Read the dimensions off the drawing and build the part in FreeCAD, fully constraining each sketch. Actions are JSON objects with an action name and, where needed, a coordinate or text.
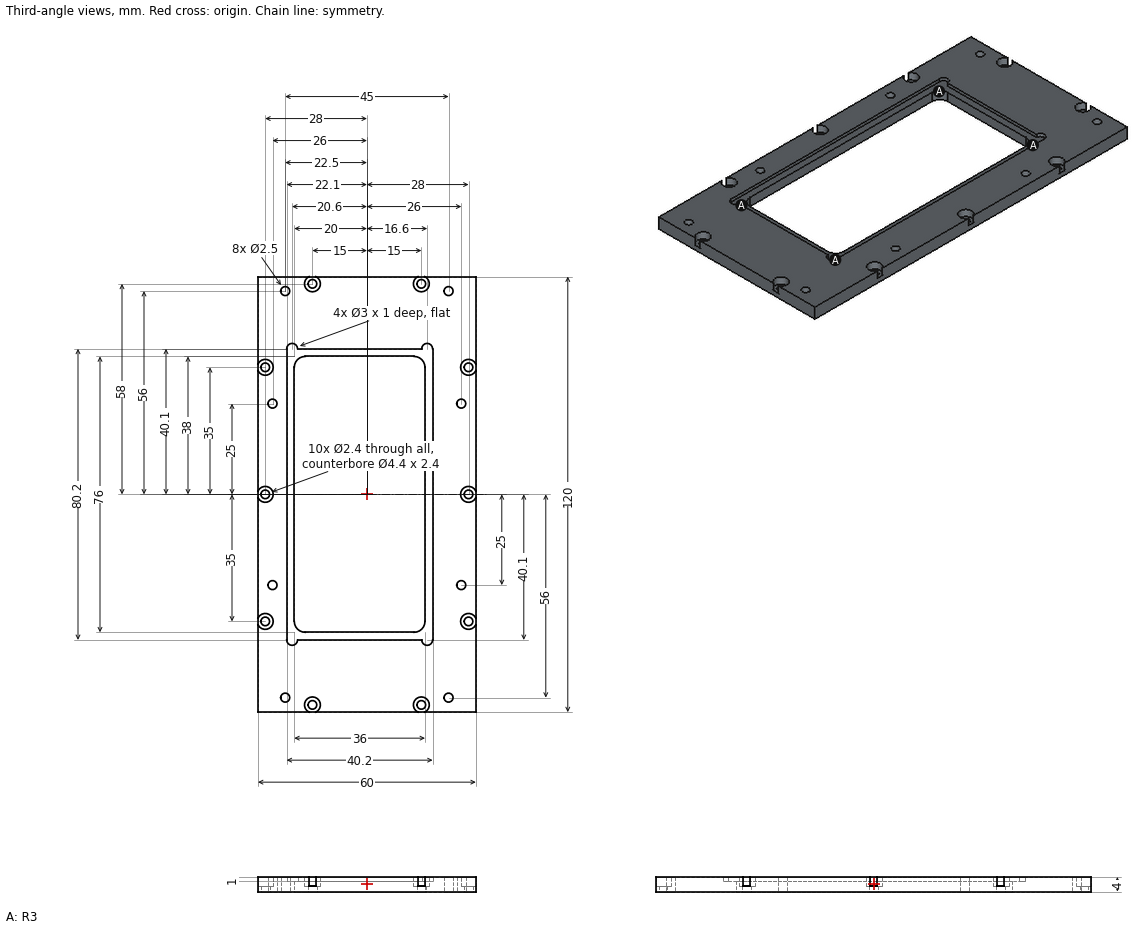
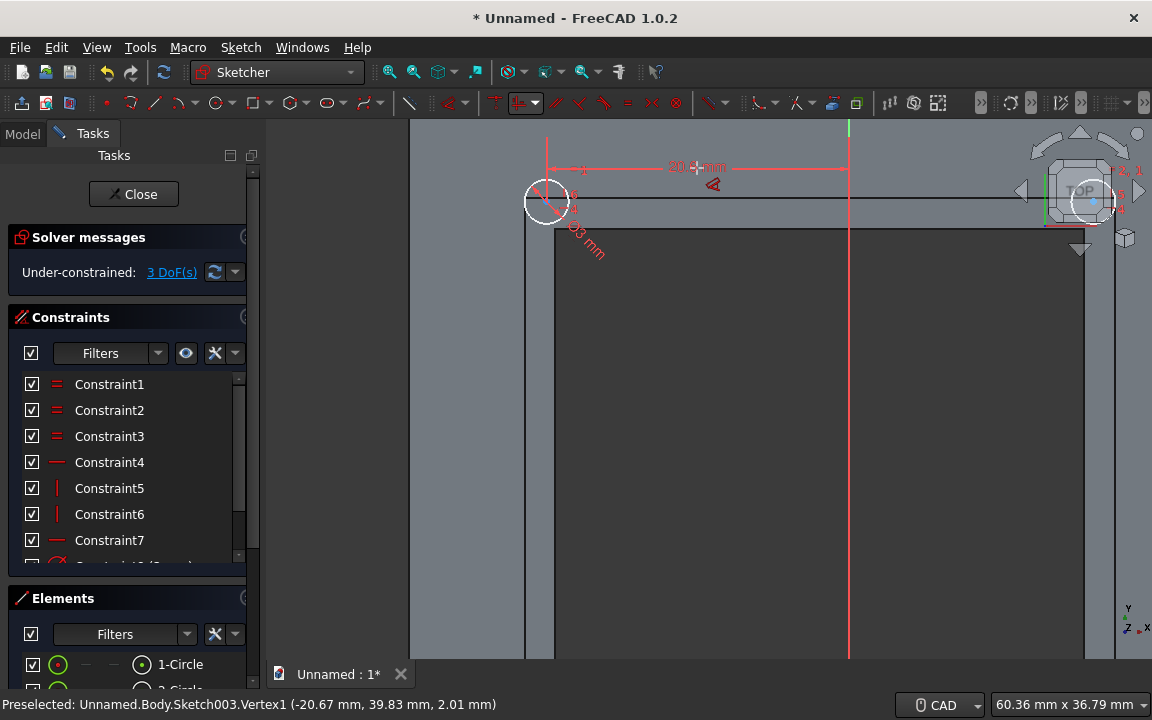
{"action": "left_click", "coordinate": [547, 202]}
{"action": "left_click", "coordinate": [513, 416]}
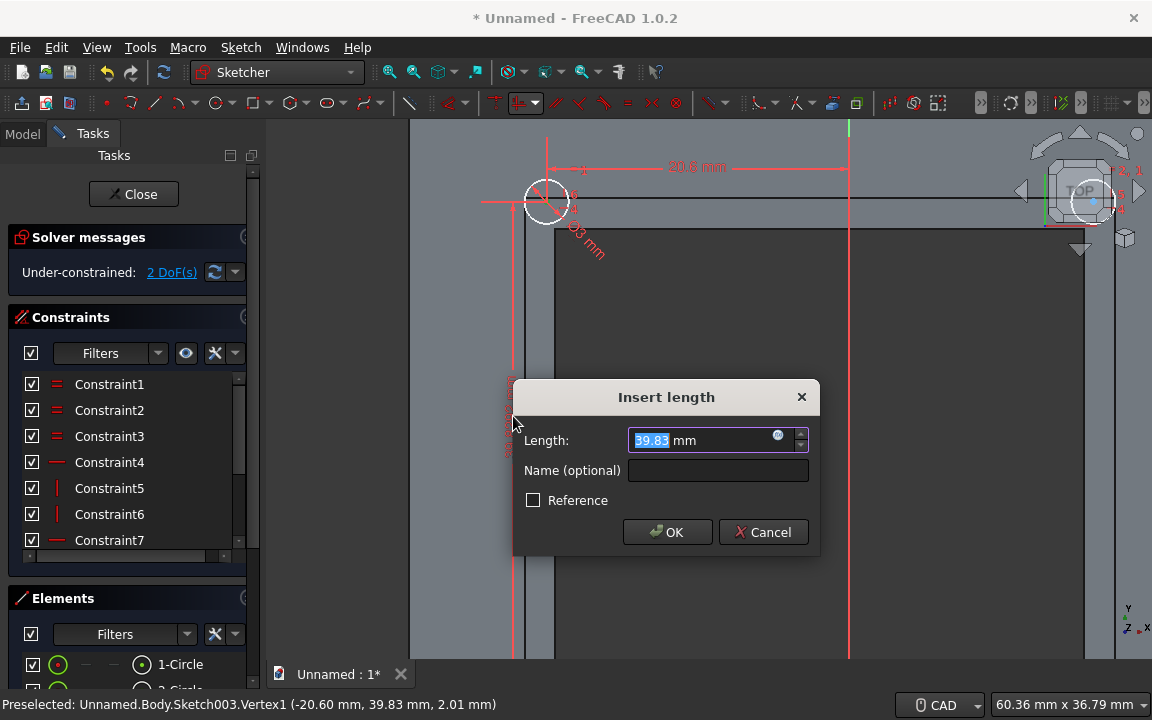
{"action": "type", "text": "40.1"}
{"action": "key", "text": "Return"}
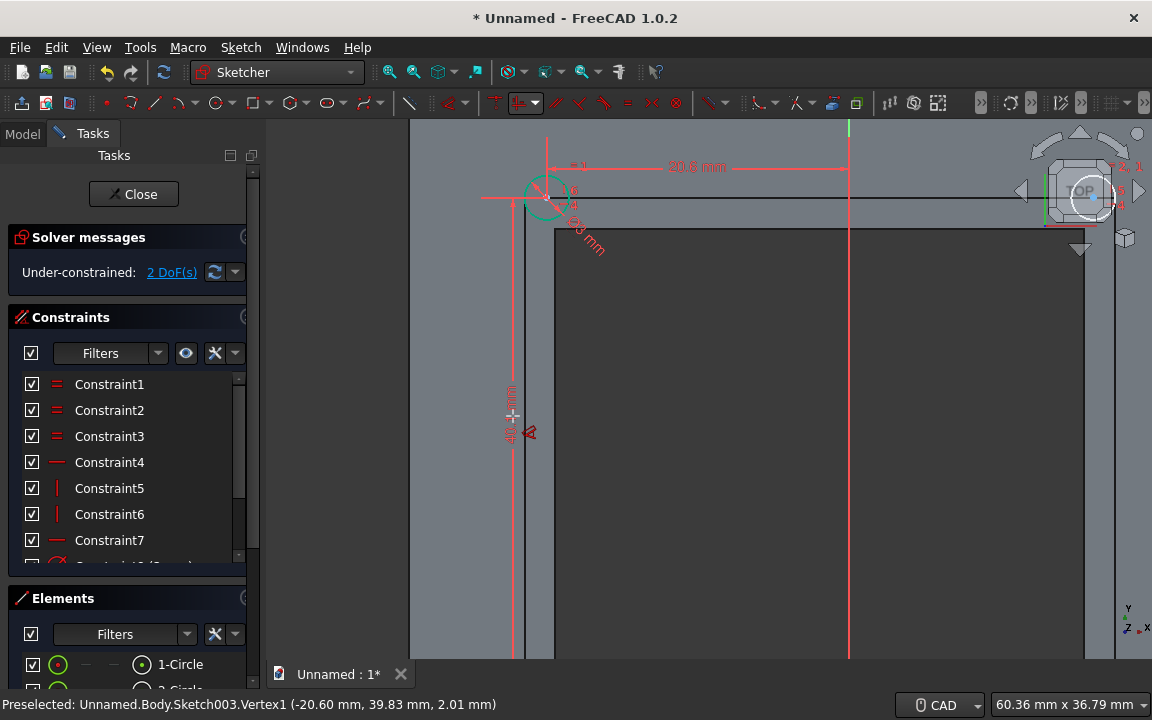
{"action": "scroll", "coordinate": [563, 218], "scroll_direction": "down", "scroll_amount": 6}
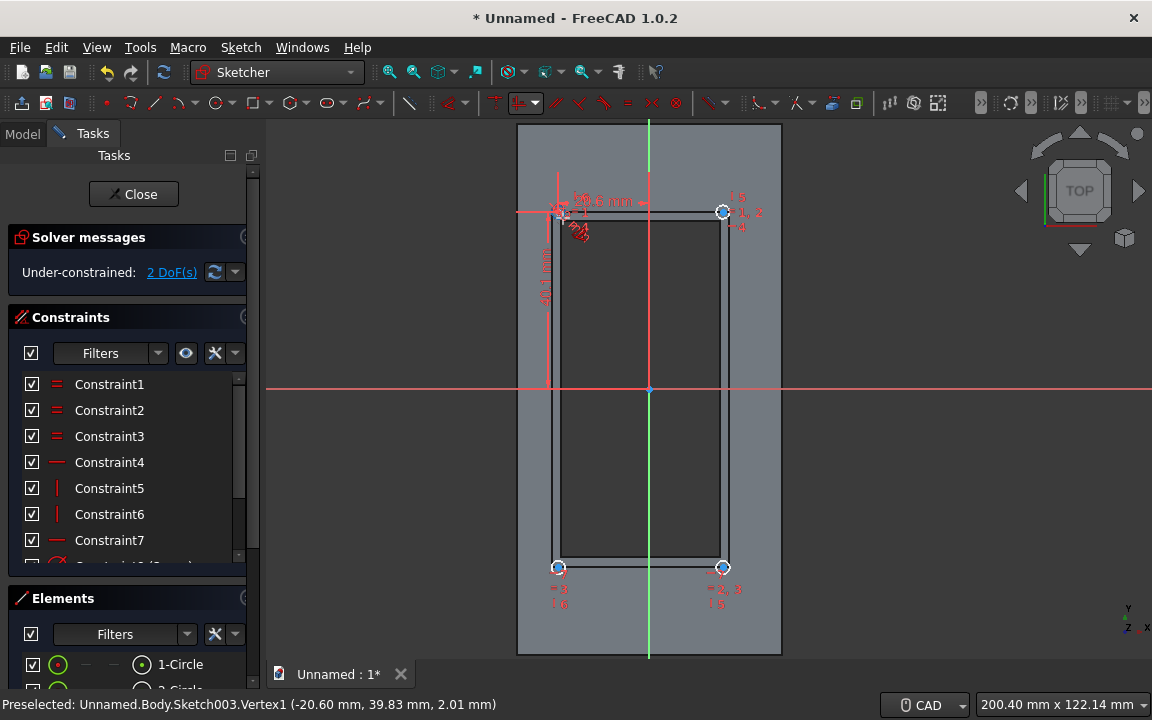
{"action": "left_click", "coordinate": [723, 212]}
{"action": "left_click", "coordinate": [686, 178]}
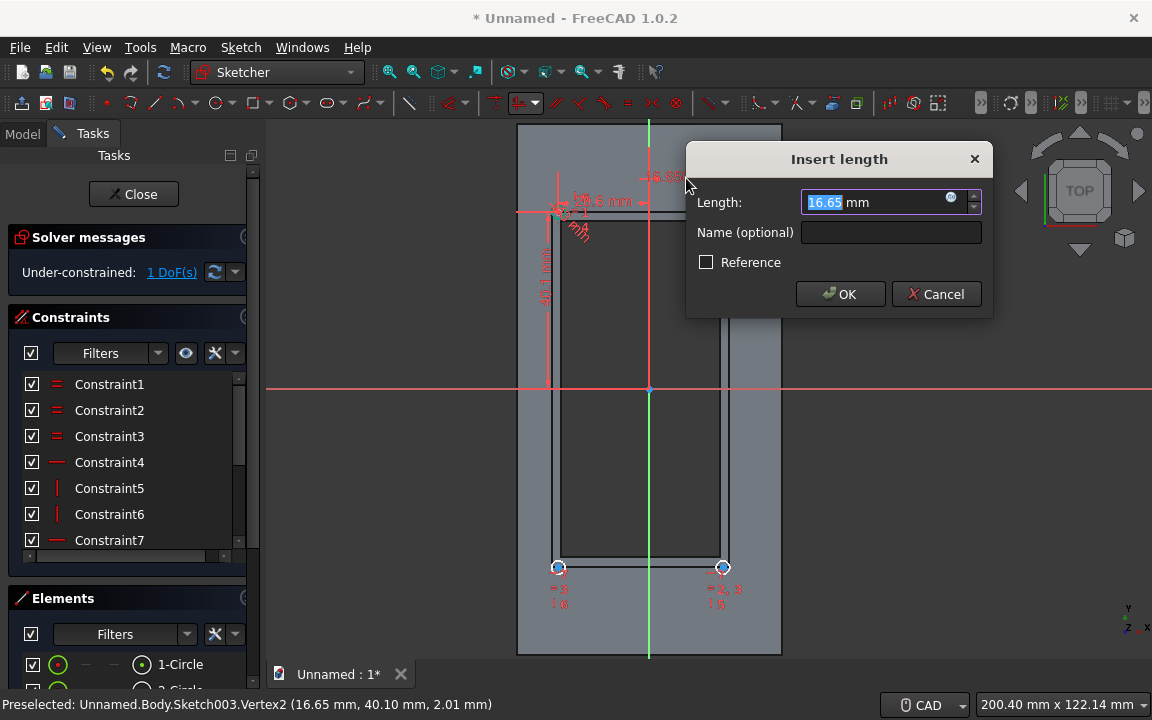
{"action": "type", "text": "16.6"}
{"action": "key", "text": "Return"}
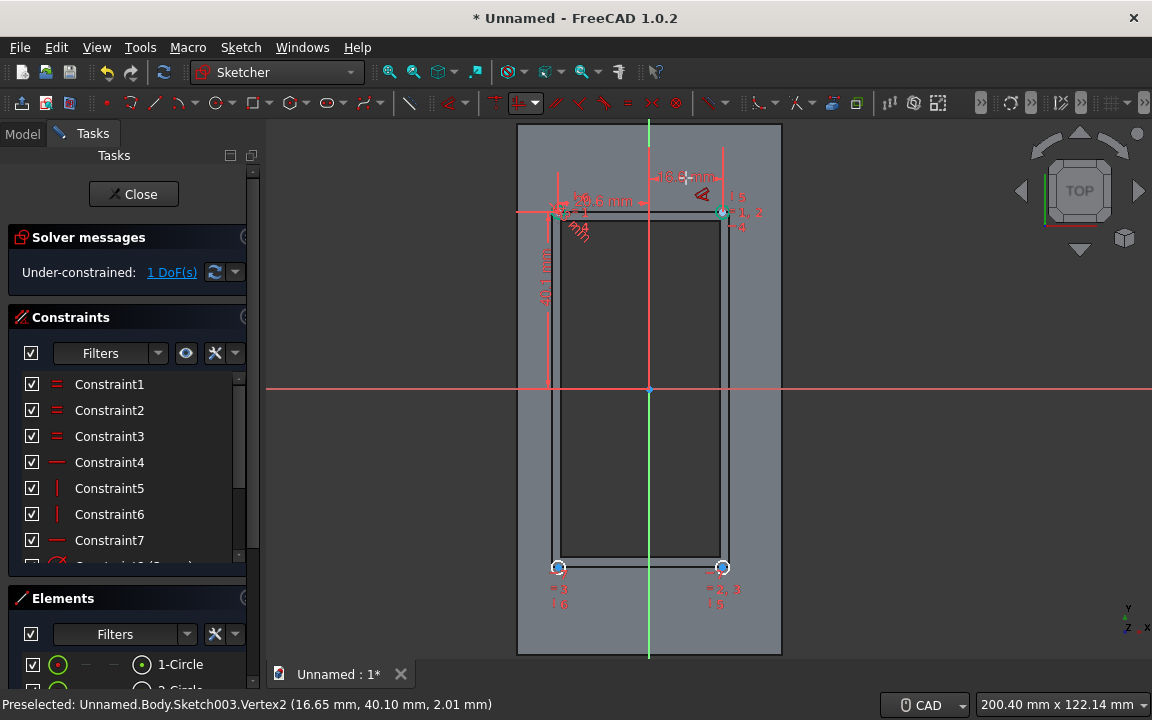
{"action": "left_click", "coordinate": [723, 567]}
{"action": "left_click", "coordinate": [757, 478]}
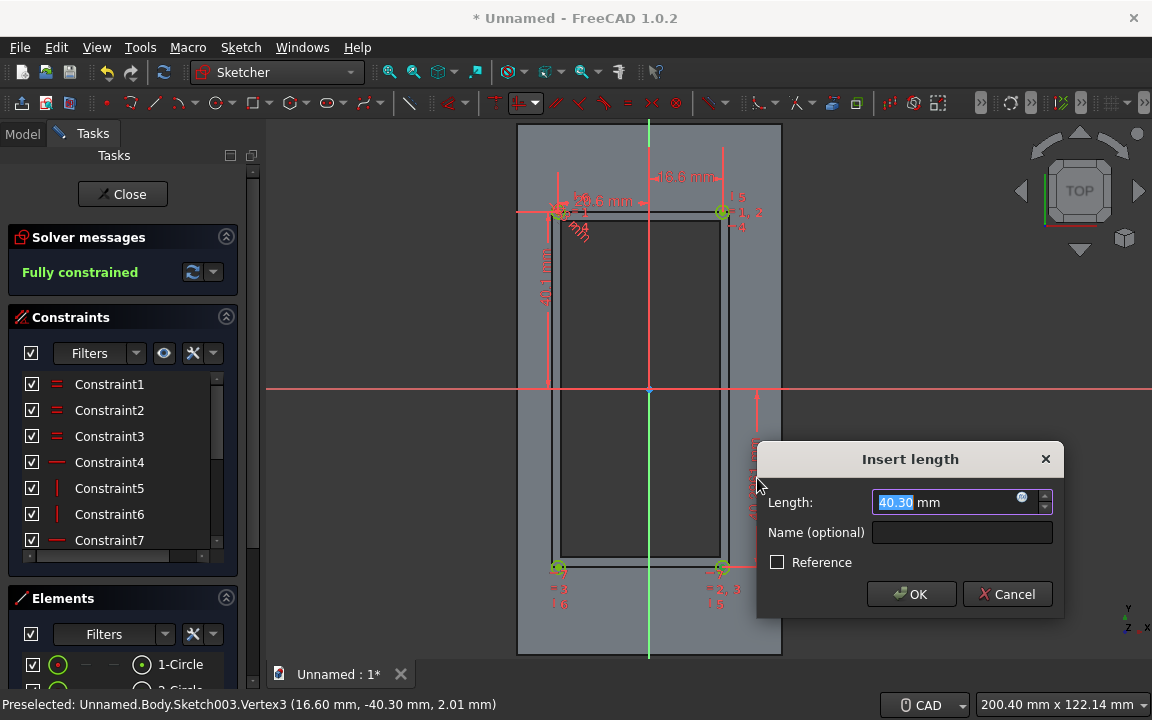
{"action": "type", "text": "40.1"}
{"action": "key", "text": "Return"}
{"action": "key", "text": "Escape"}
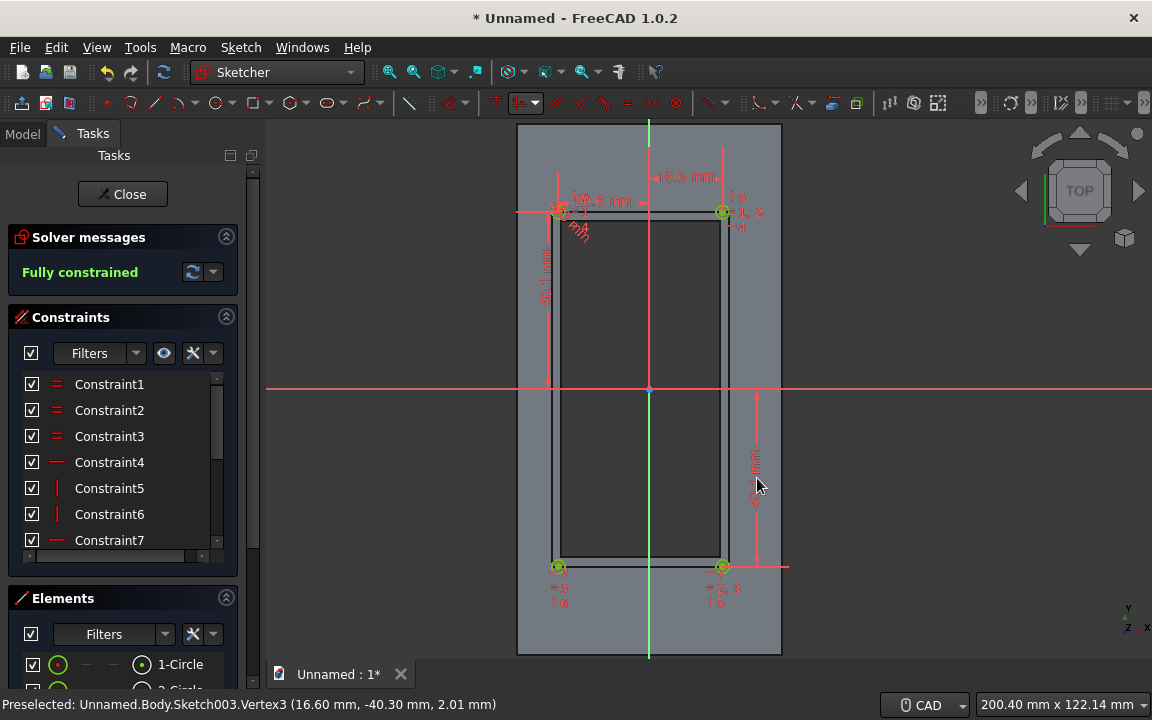
{"action": "left_click", "coordinate": [123, 194]}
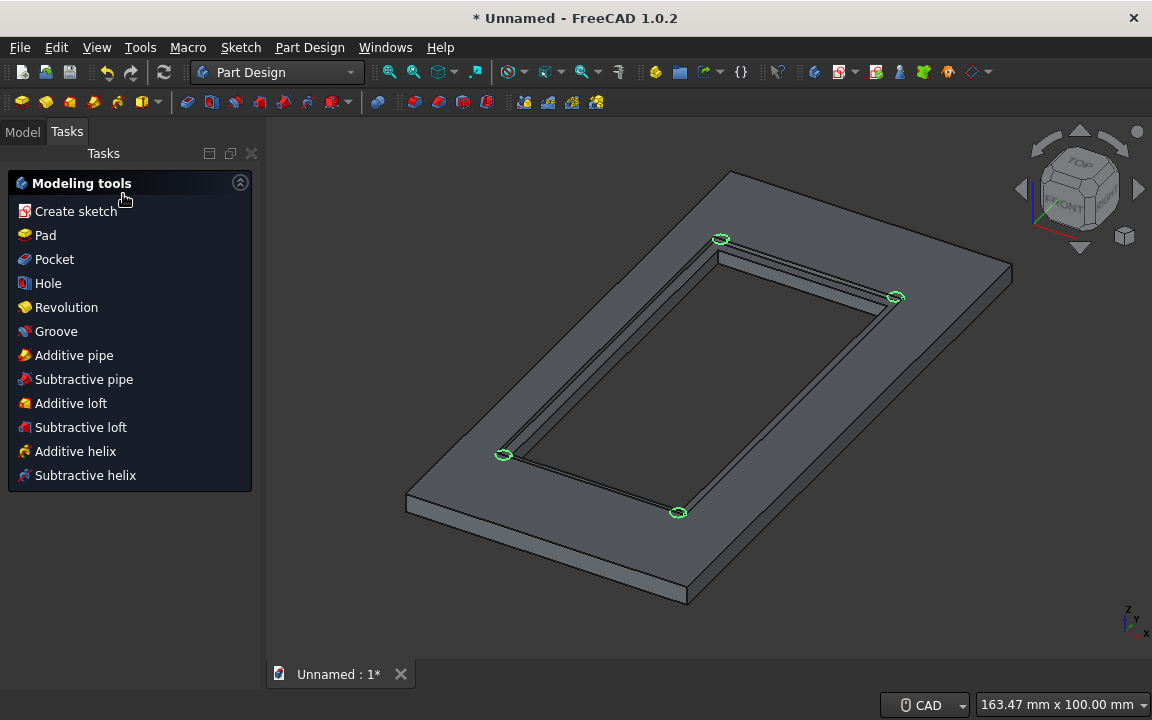
{"action": "left_click", "coordinate": [212, 102]}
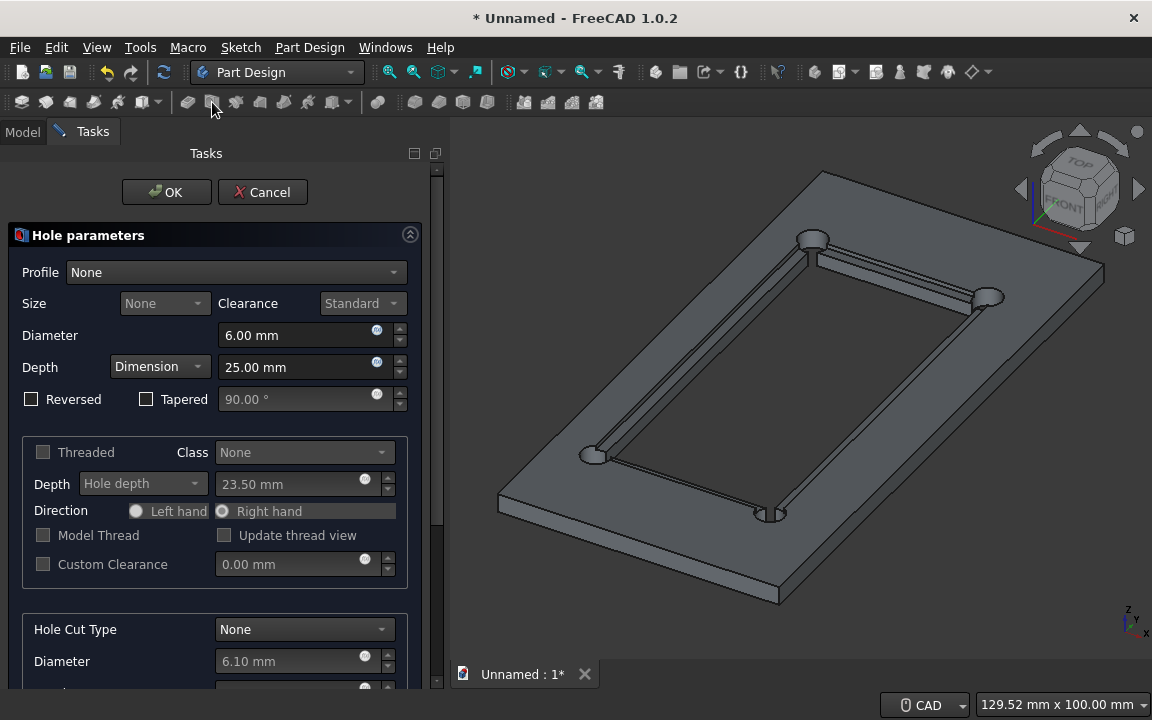
{"action": "triple_click", "coordinate": [305, 335]}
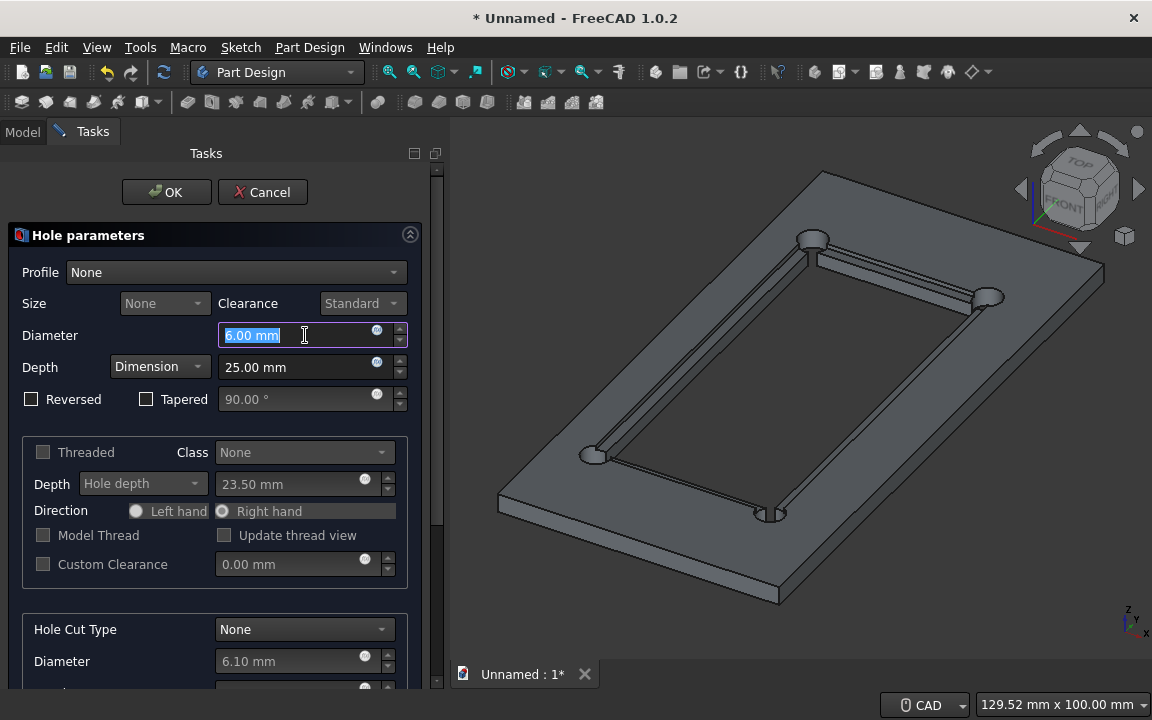
{"action": "type", "text": "3"}
{"action": "key", "text": "Tab"}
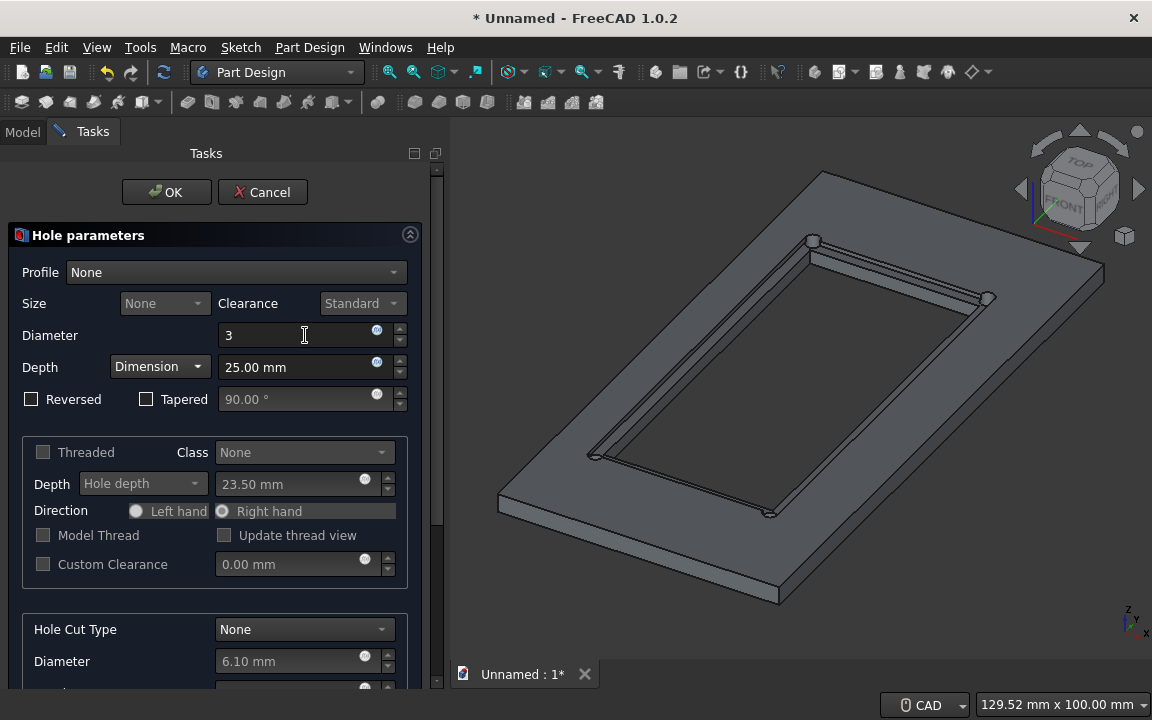
{"action": "triple_click", "coordinate": [305, 367]}